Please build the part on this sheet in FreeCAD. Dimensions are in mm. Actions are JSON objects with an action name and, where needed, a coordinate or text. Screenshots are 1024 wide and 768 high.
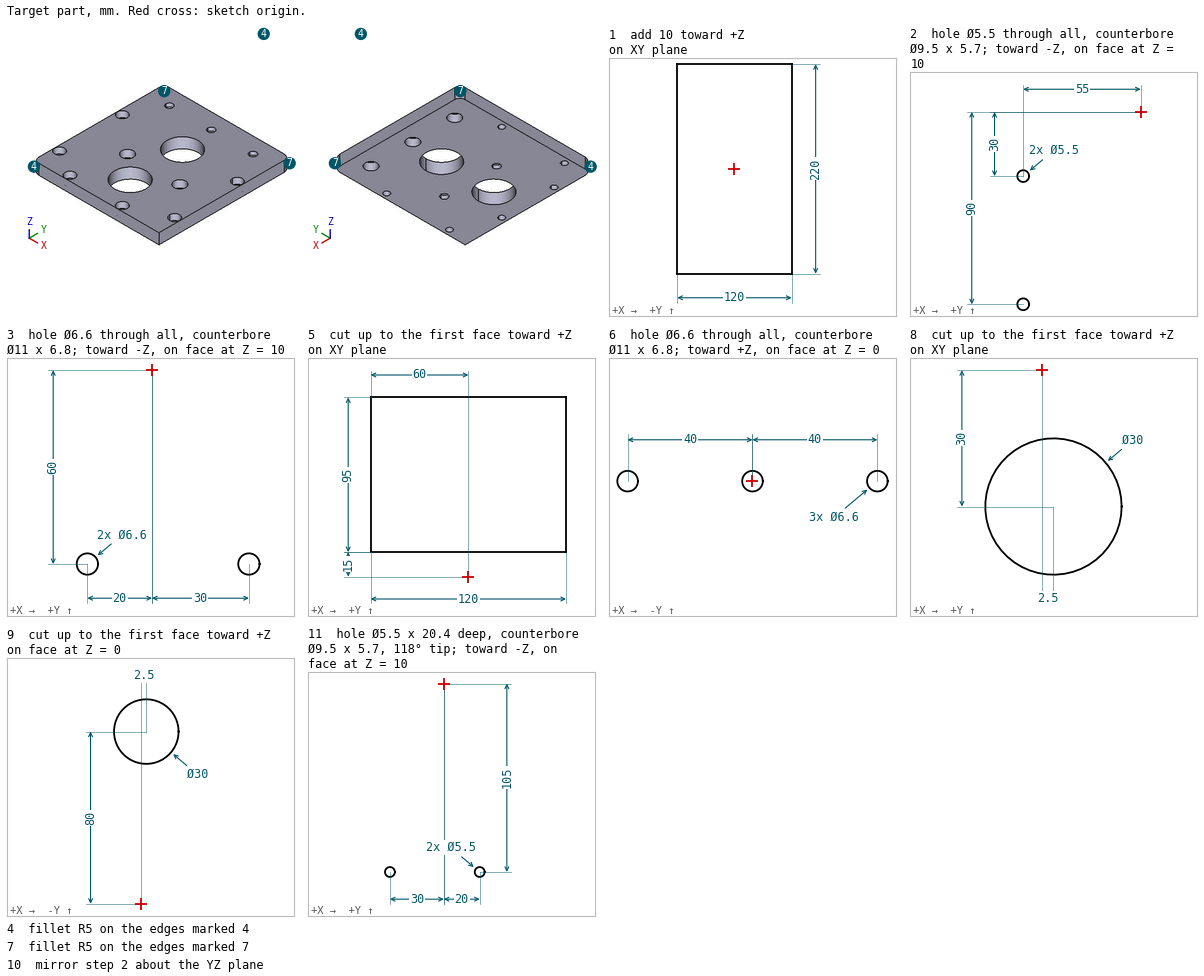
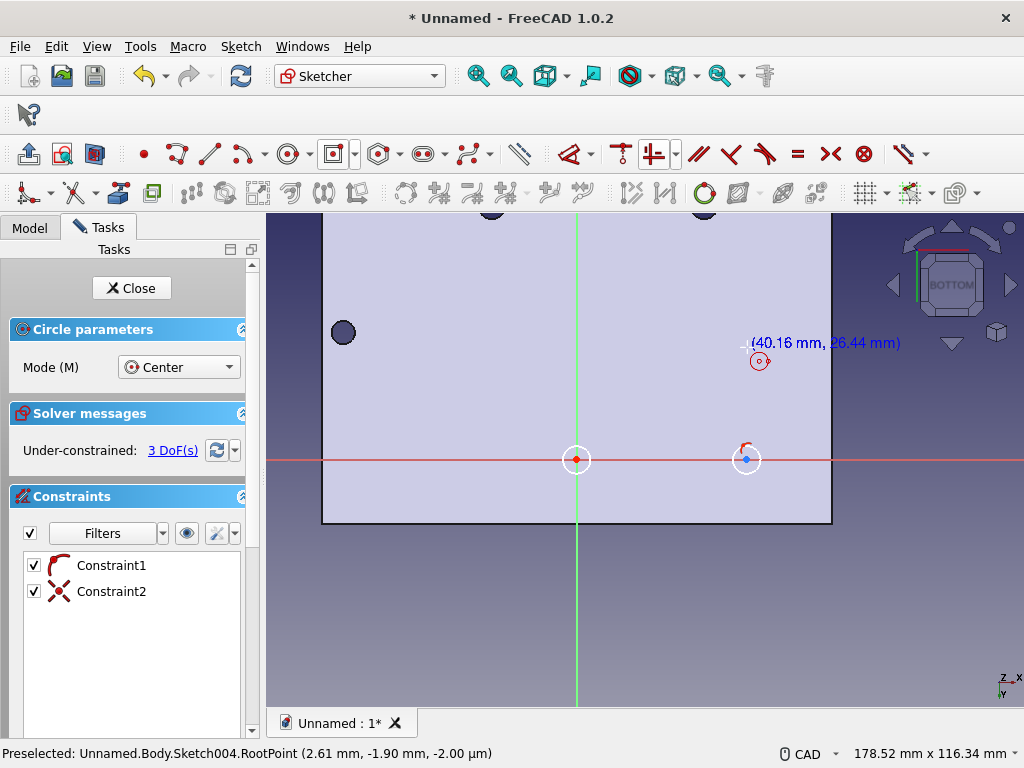
{"action": "scroll", "coordinate": [407, 460], "scroll_direction": "up", "scroll_amount": 3}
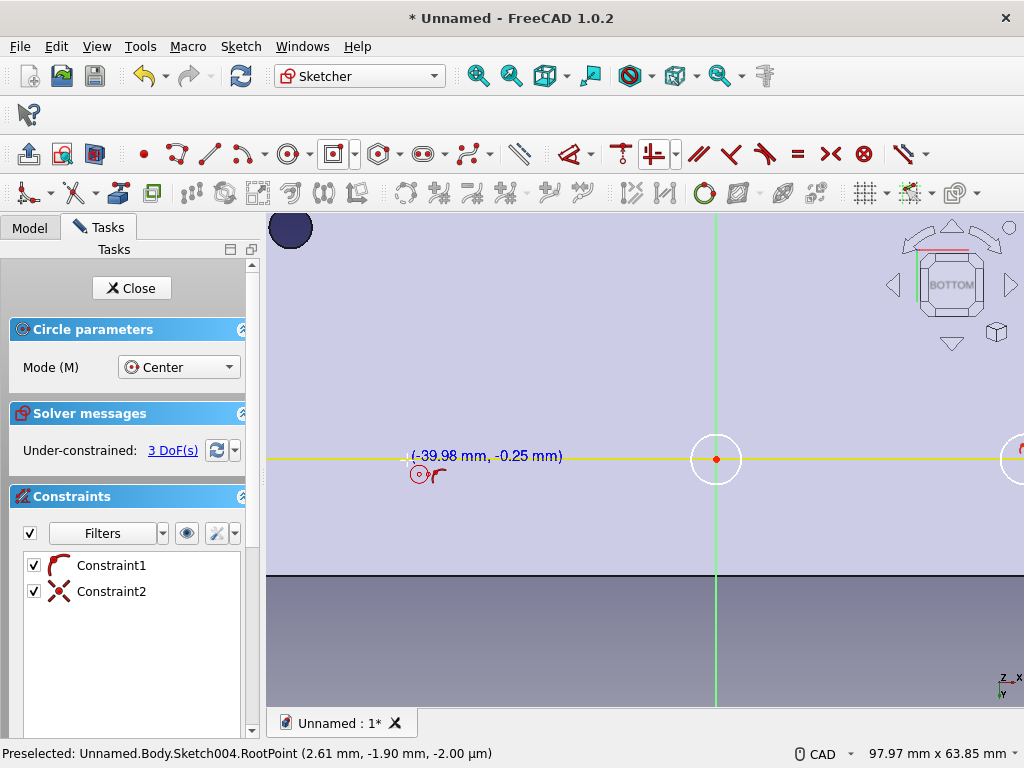
{"action": "left_click", "coordinate": [407, 459]}
{"action": "left_click", "coordinate": [425, 441]}
{"action": "key", "text": "Escape"}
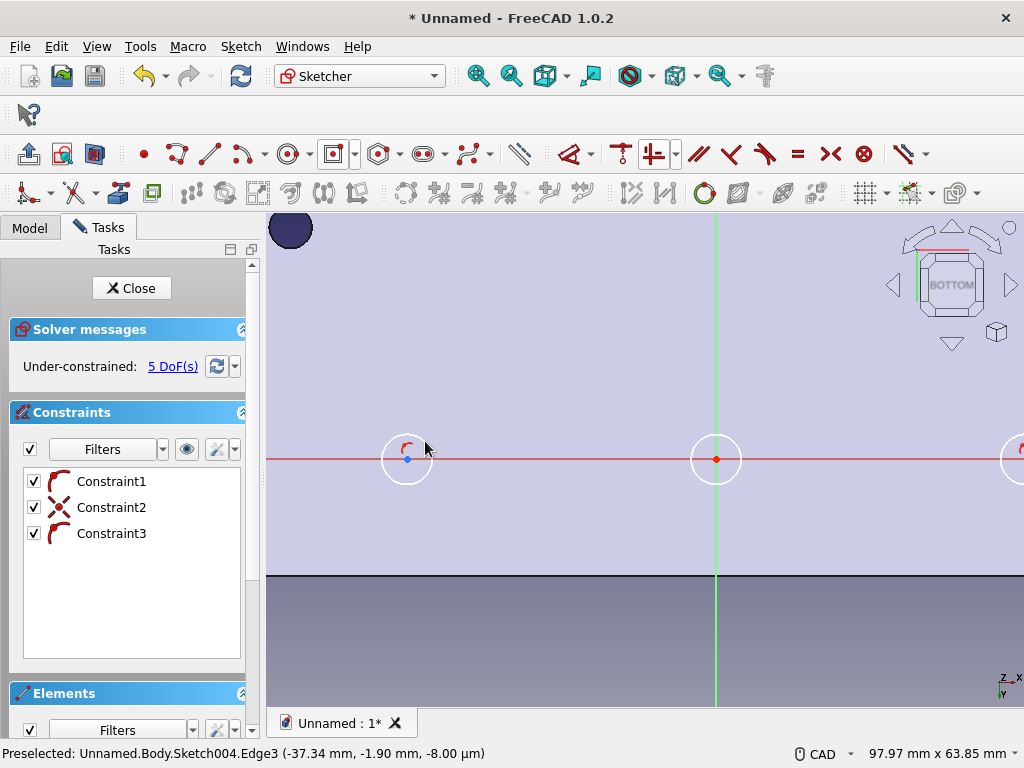
{"action": "scroll", "coordinate": [407, 461], "scroll_direction": "down", "scroll_amount": 3}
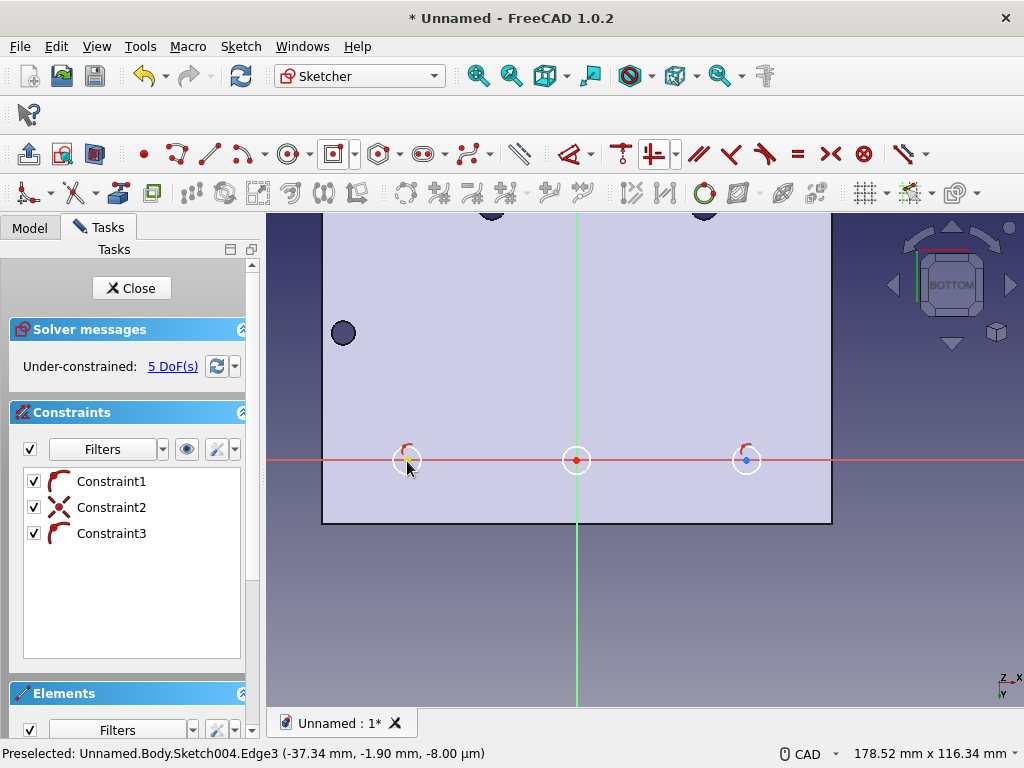
{"action": "scroll", "coordinate": [756, 451], "scroll_direction": "up", "scroll_amount": 2}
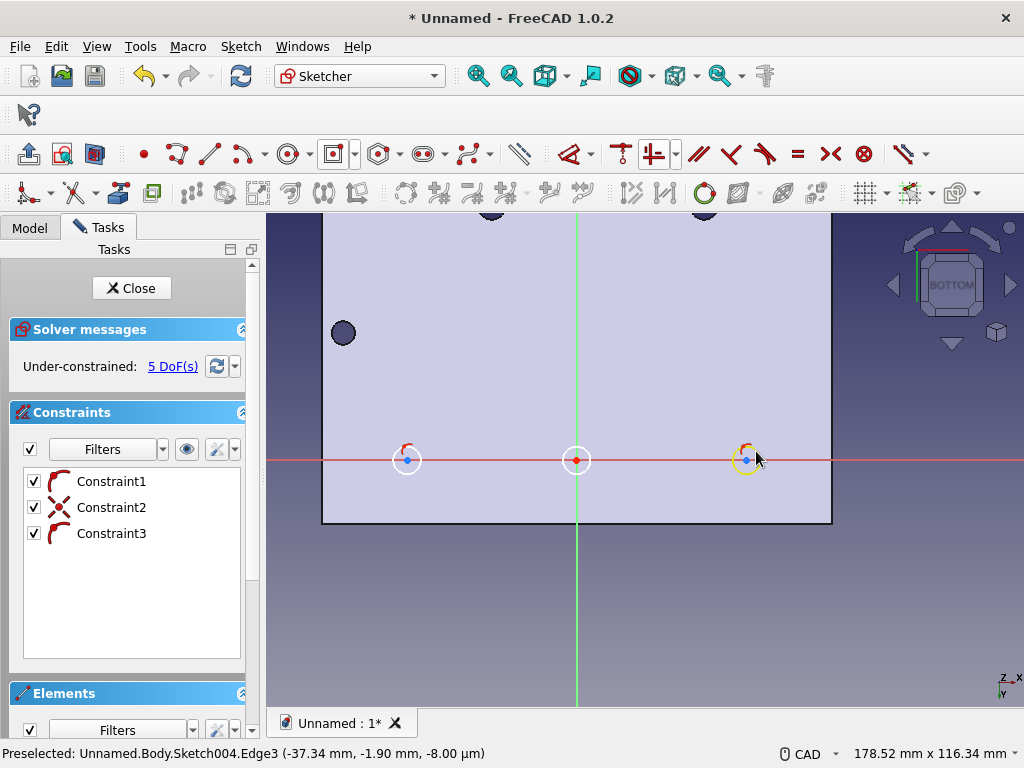
{"action": "left_click", "coordinate": [756, 450]}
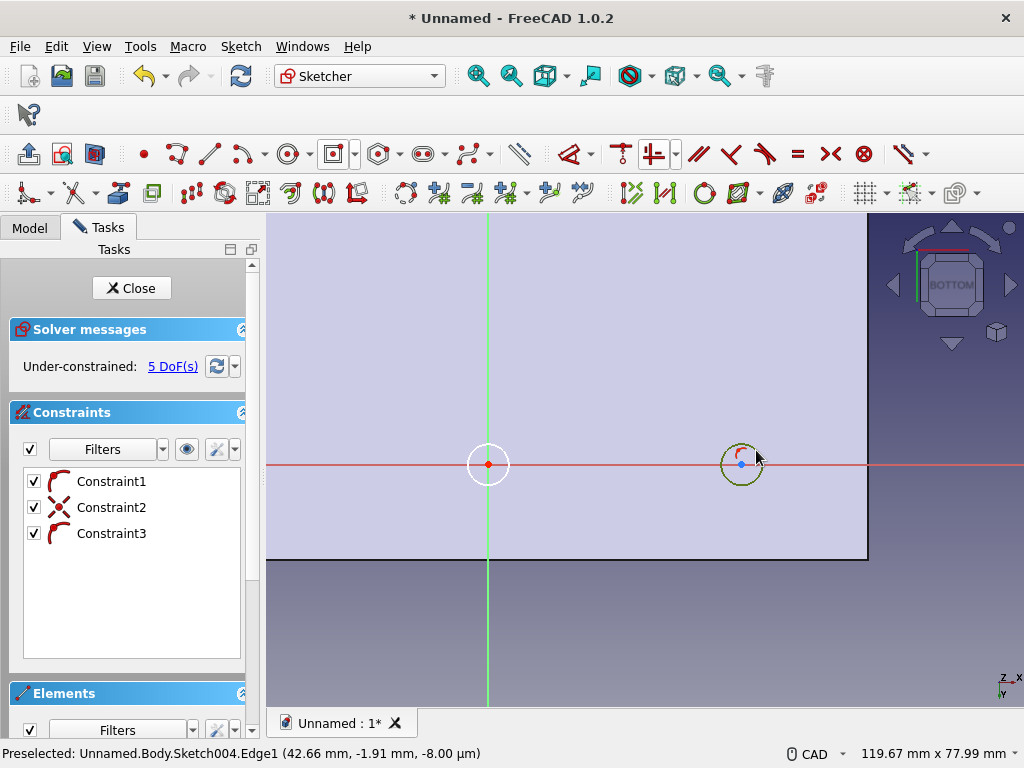
{"action": "left_click", "coordinate": [503, 450]}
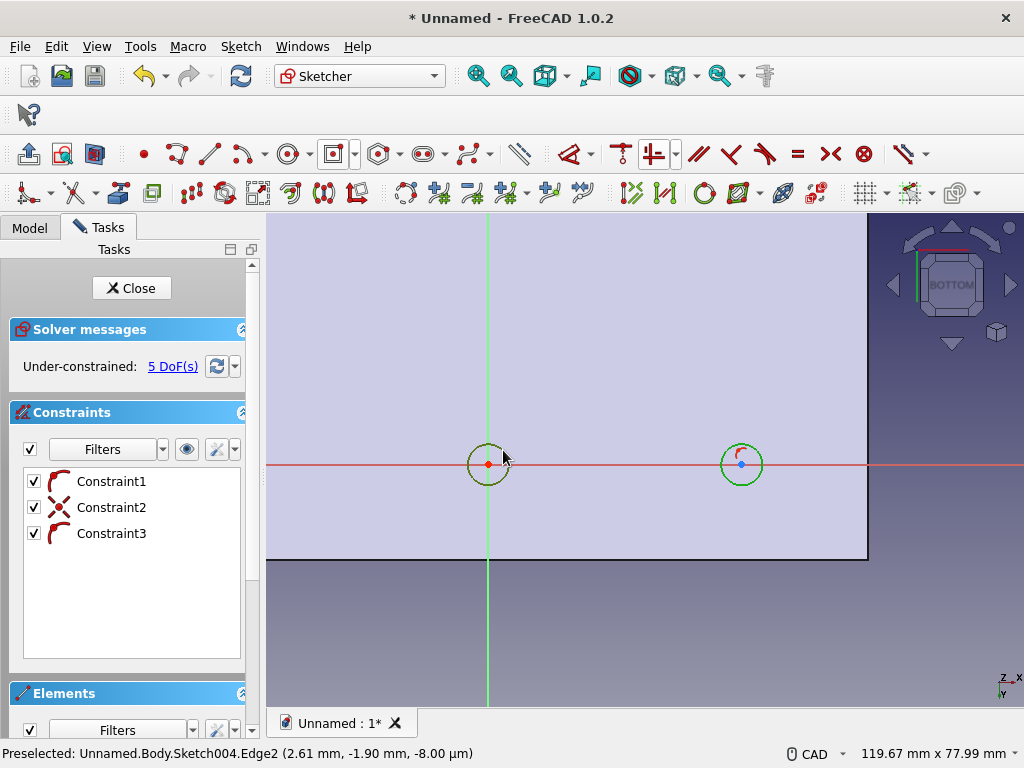
{"action": "scroll", "coordinate": [756, 450], "scroll_direction": "down", "scroll_amount": 2}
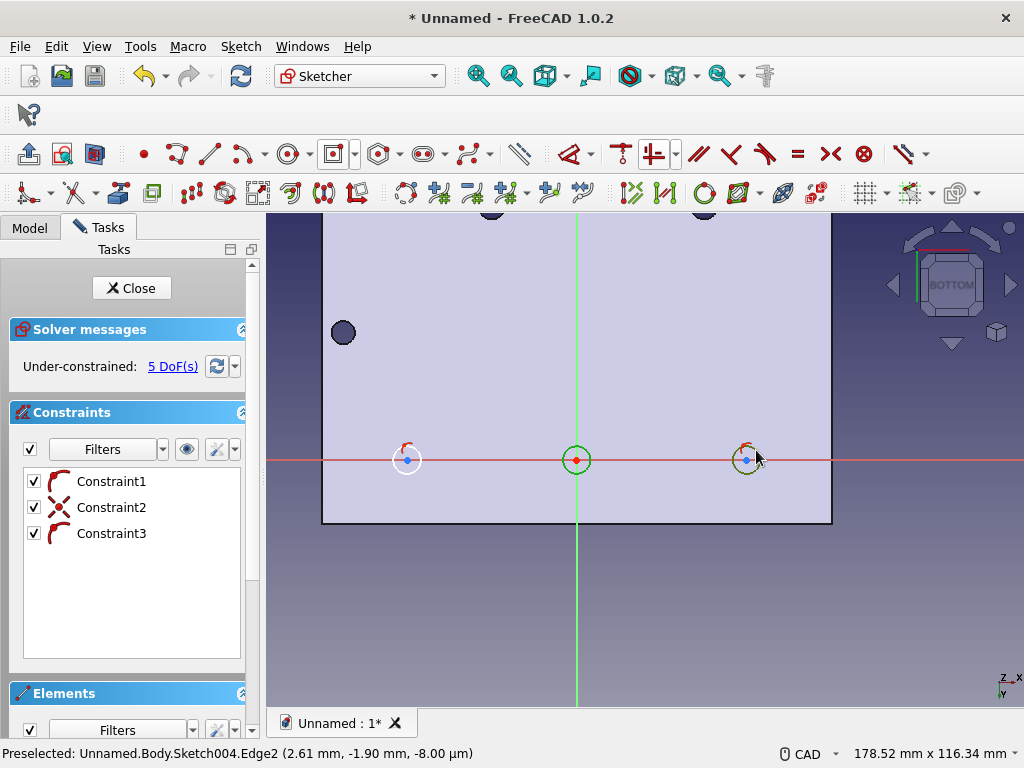
{"action": "scroll", "coordinate": [417, 450], "scroll_direction": "up", "scroll_amount": 2}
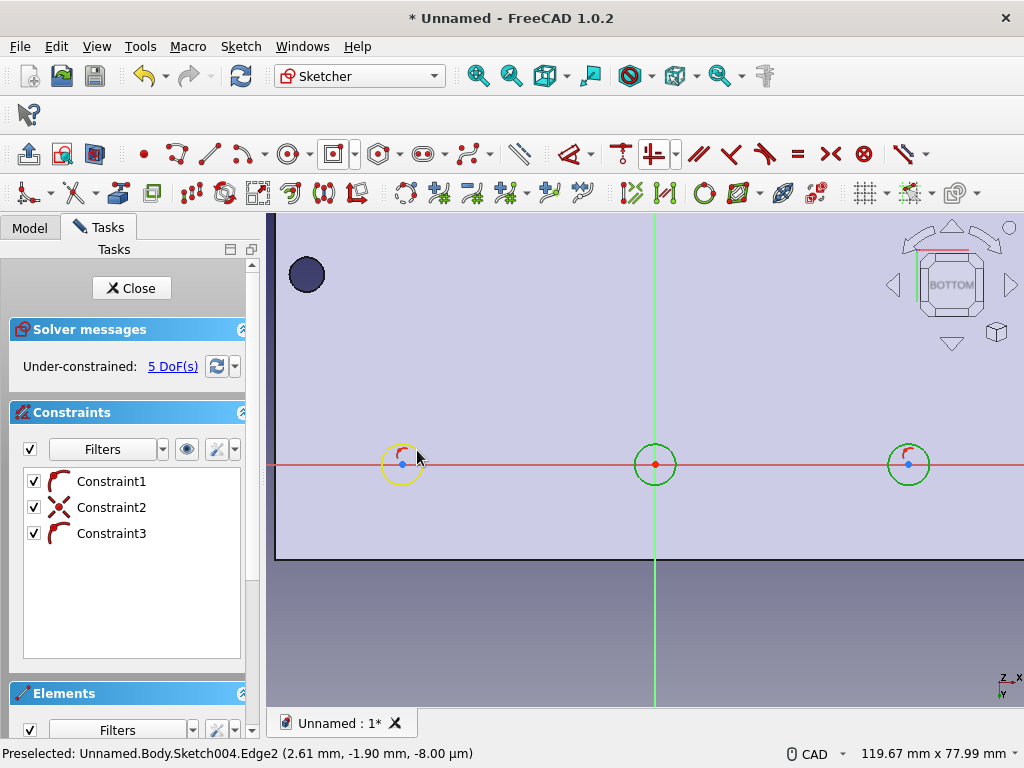
{"action": "left_click", "coordinate": [417, 450]}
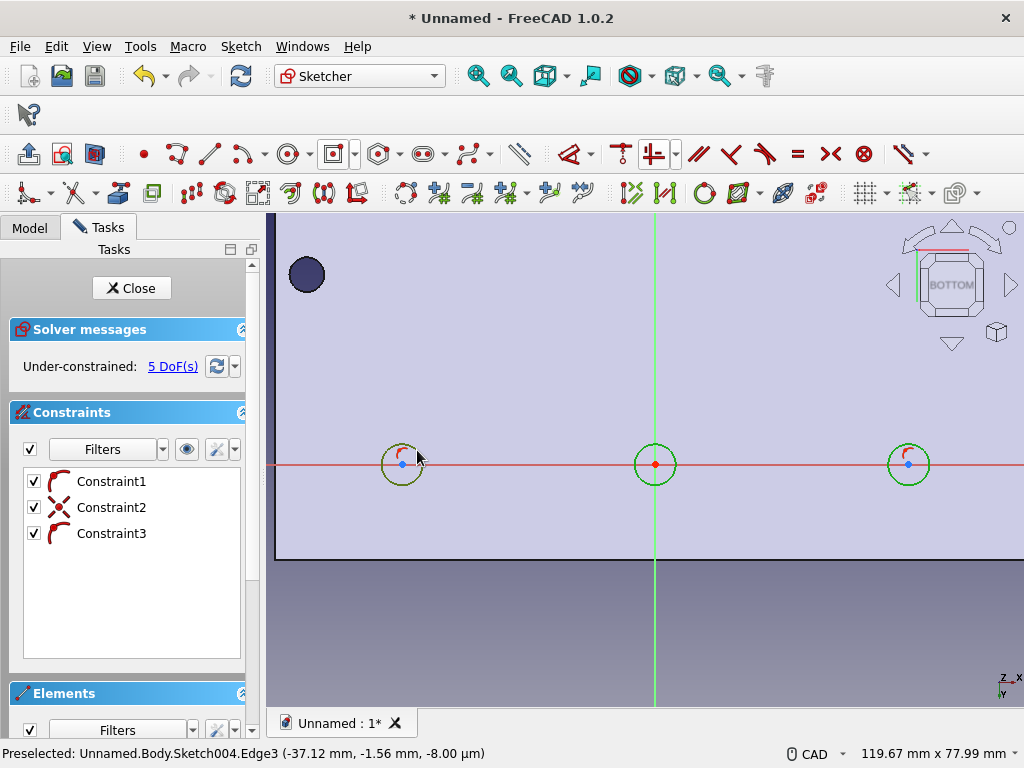
{"action": "key", "text": "e"}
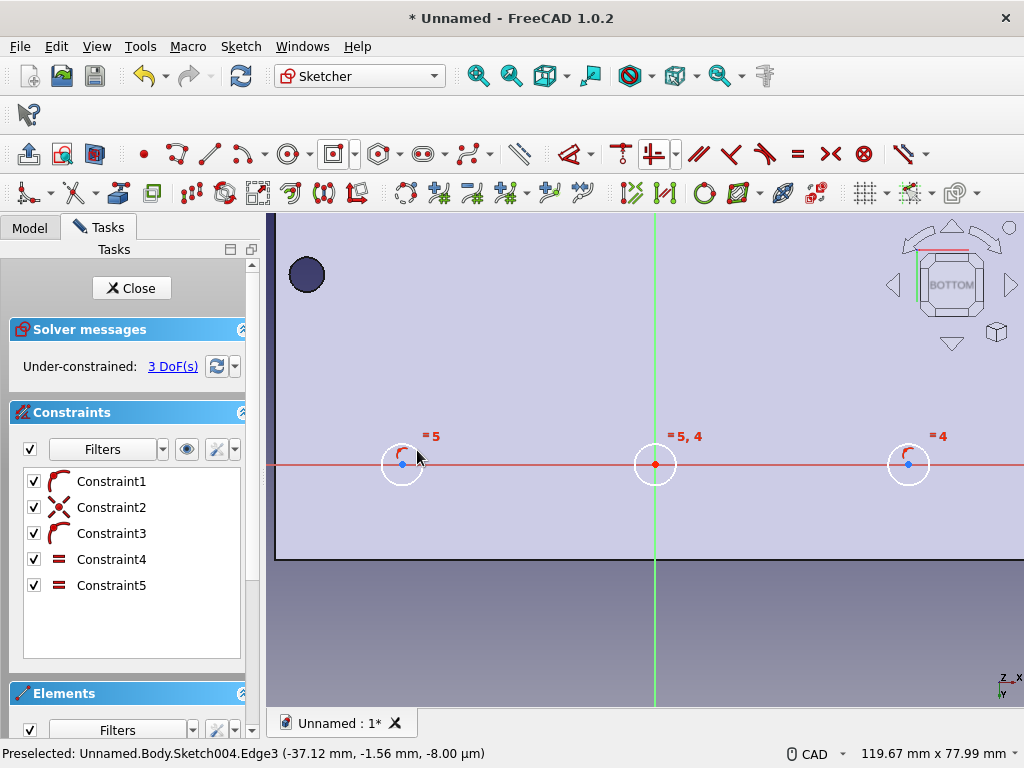
{"action": "left_click", "coordinate": [568, 154]}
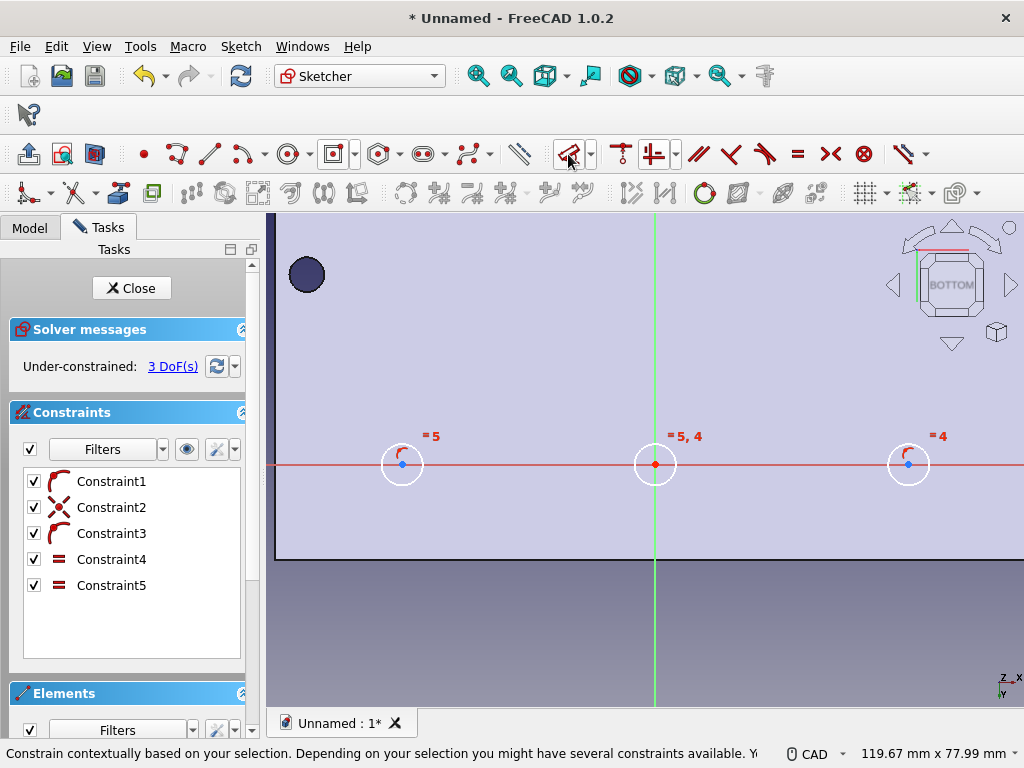
{"action": "scroll", "coordinate": [416, 450], "scroll_direction": "down", "scroll_amount": 2}